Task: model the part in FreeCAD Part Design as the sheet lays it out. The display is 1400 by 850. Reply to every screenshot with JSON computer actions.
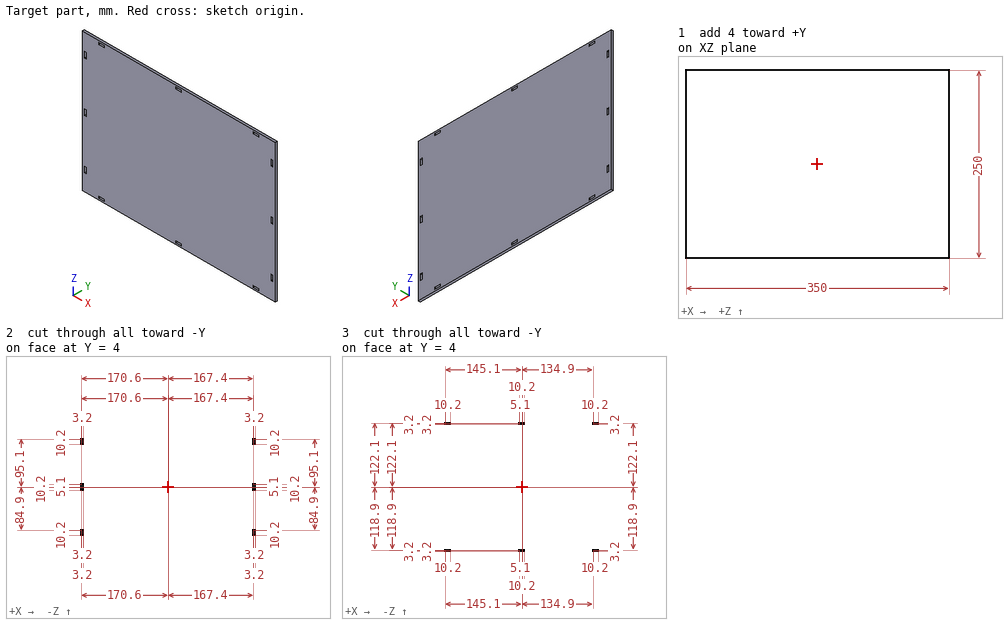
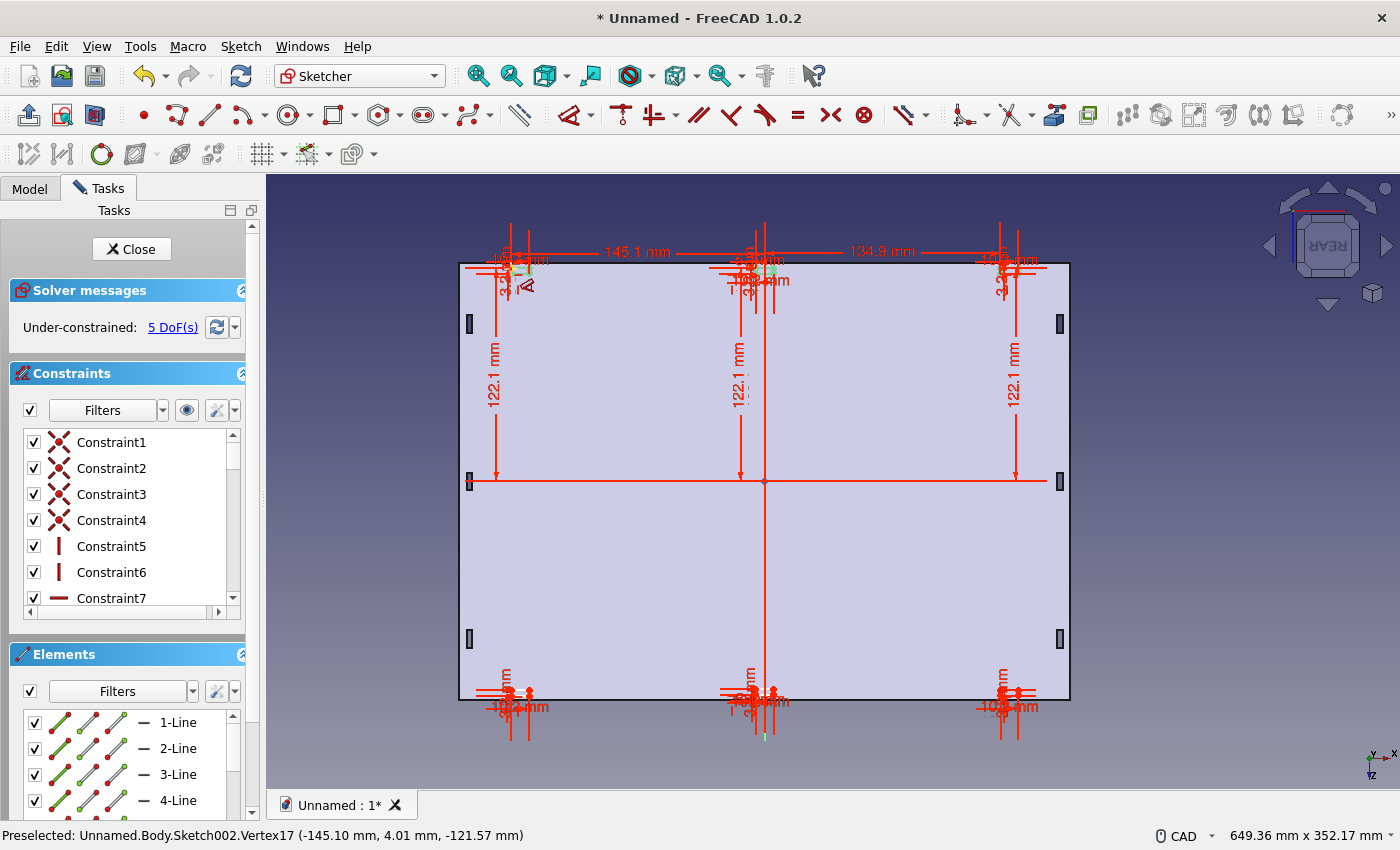
{"action": "scroll", "coordinate": [511, 690], "scroll_direction": "up", "scroll_amount": 4}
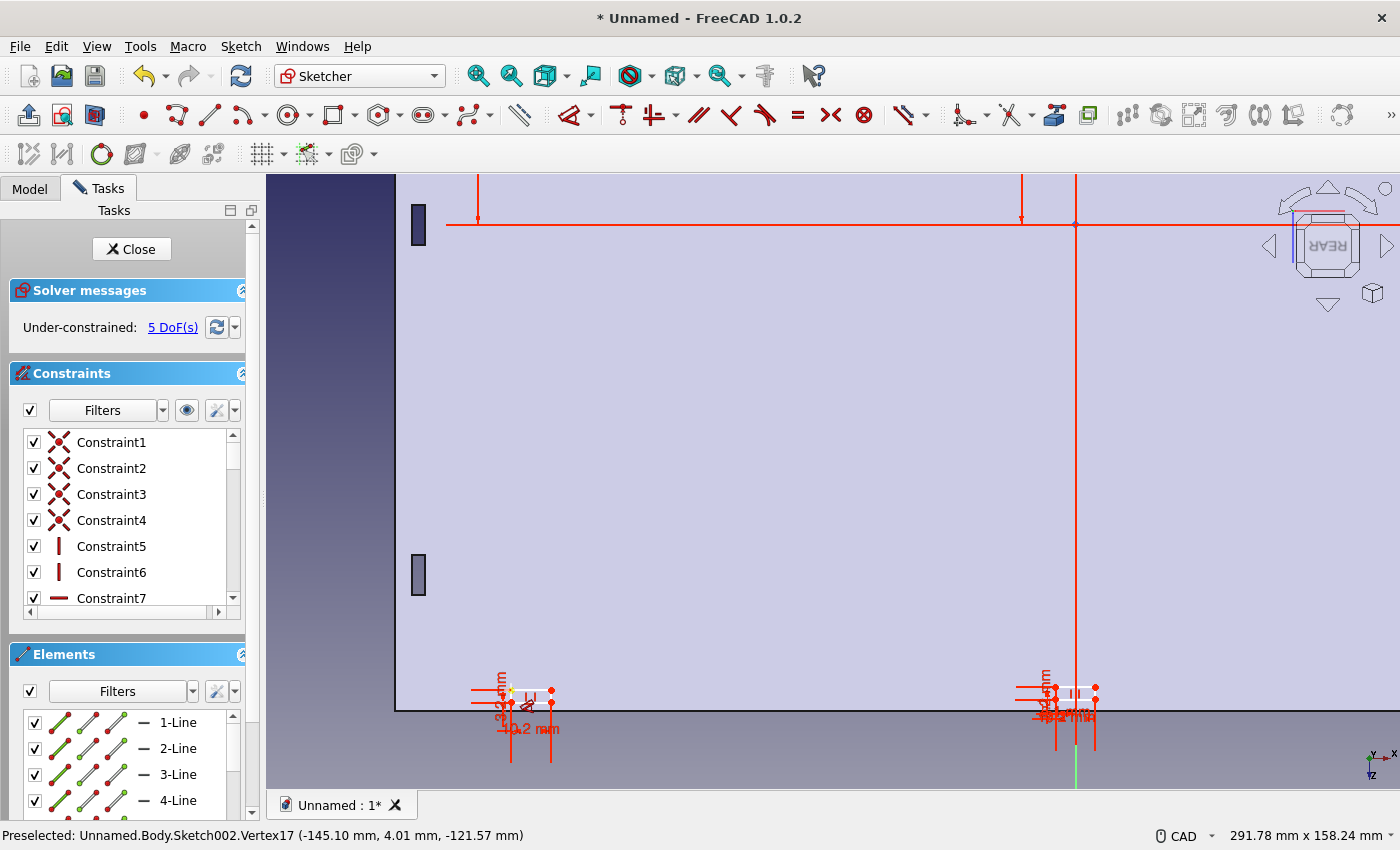
{"action": "left_click", "coordinate": [511, 690]}
{"action": "left_click", "coordinate": [793, 724]}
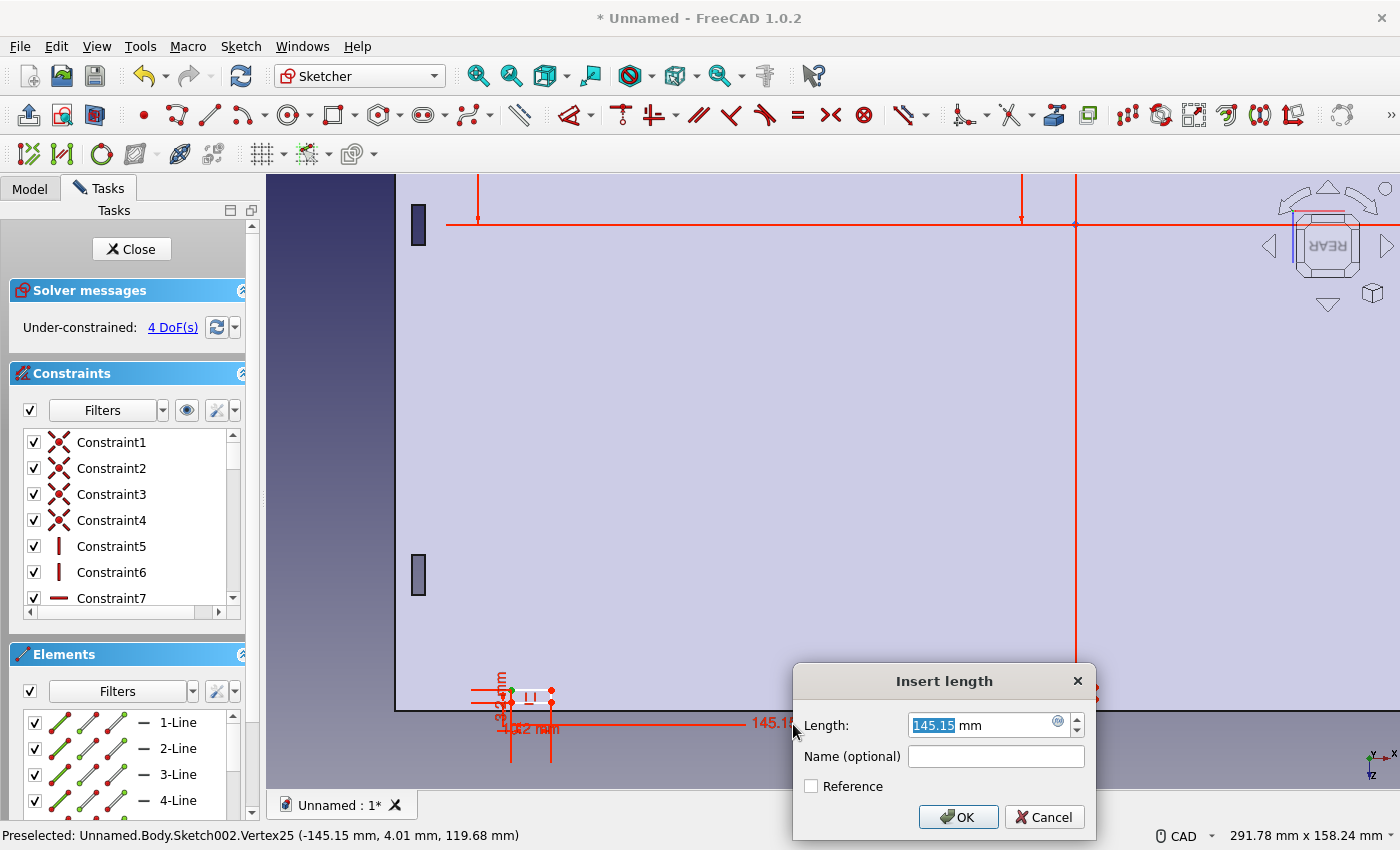
{"action": "type", "text": "145.1"}
{"action": "key", "text": "Return"}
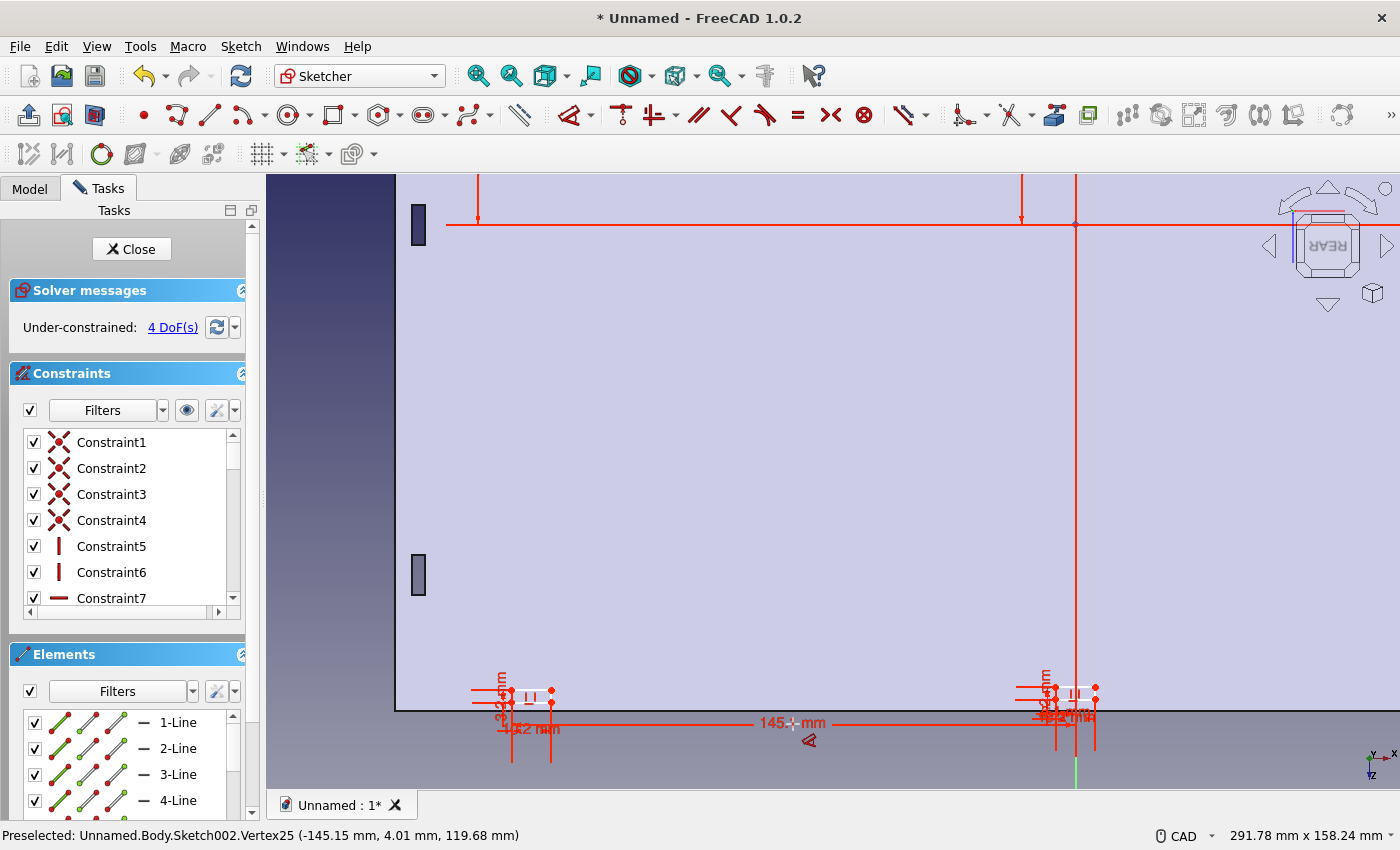
{"action": "left_click", "coordinate": [512, 690]}
{"action": "left_click", "coordinate": [478, 457]}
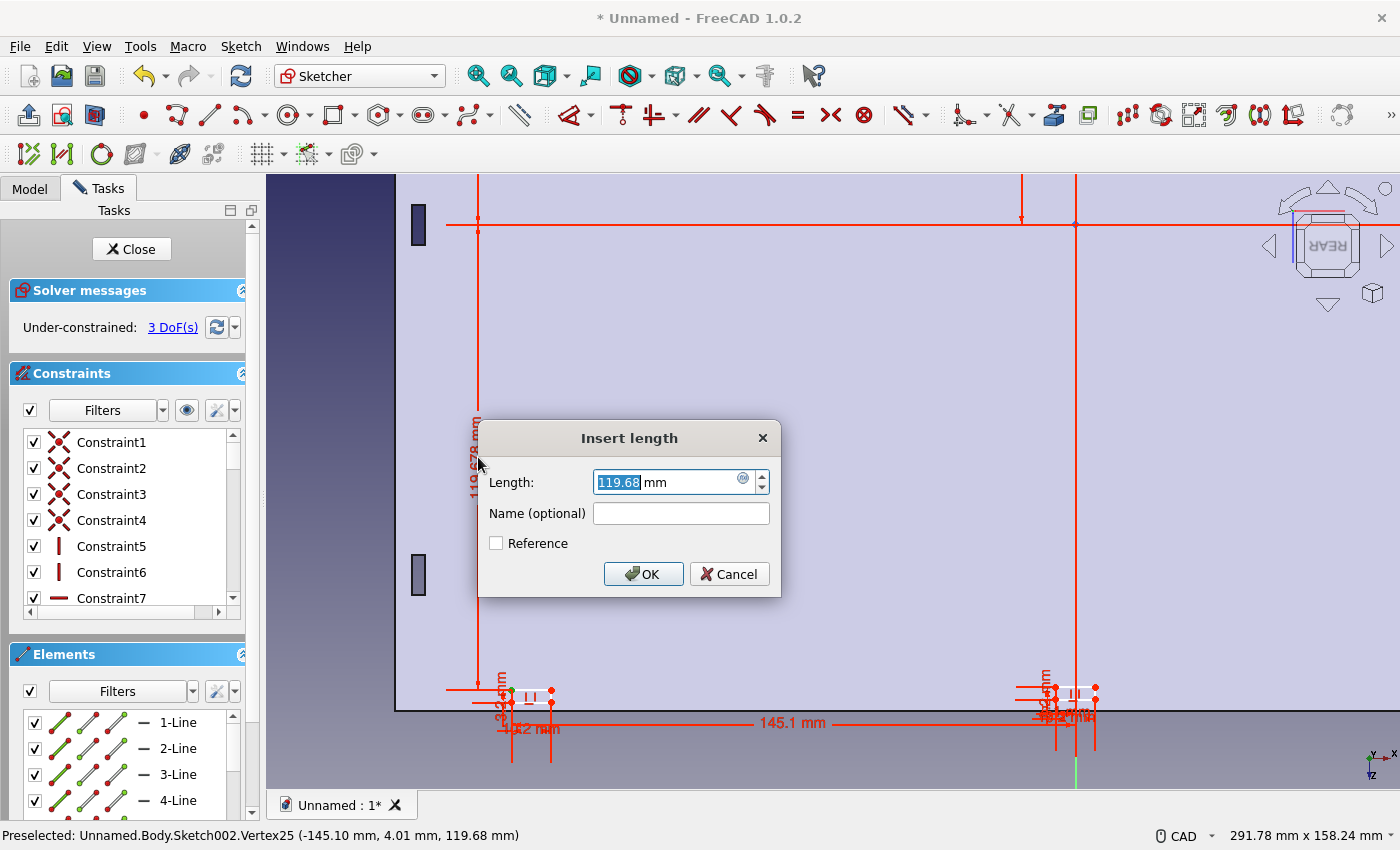
{"action": "type", "text": "118.9"}
{"action": "key", "text": "Return"}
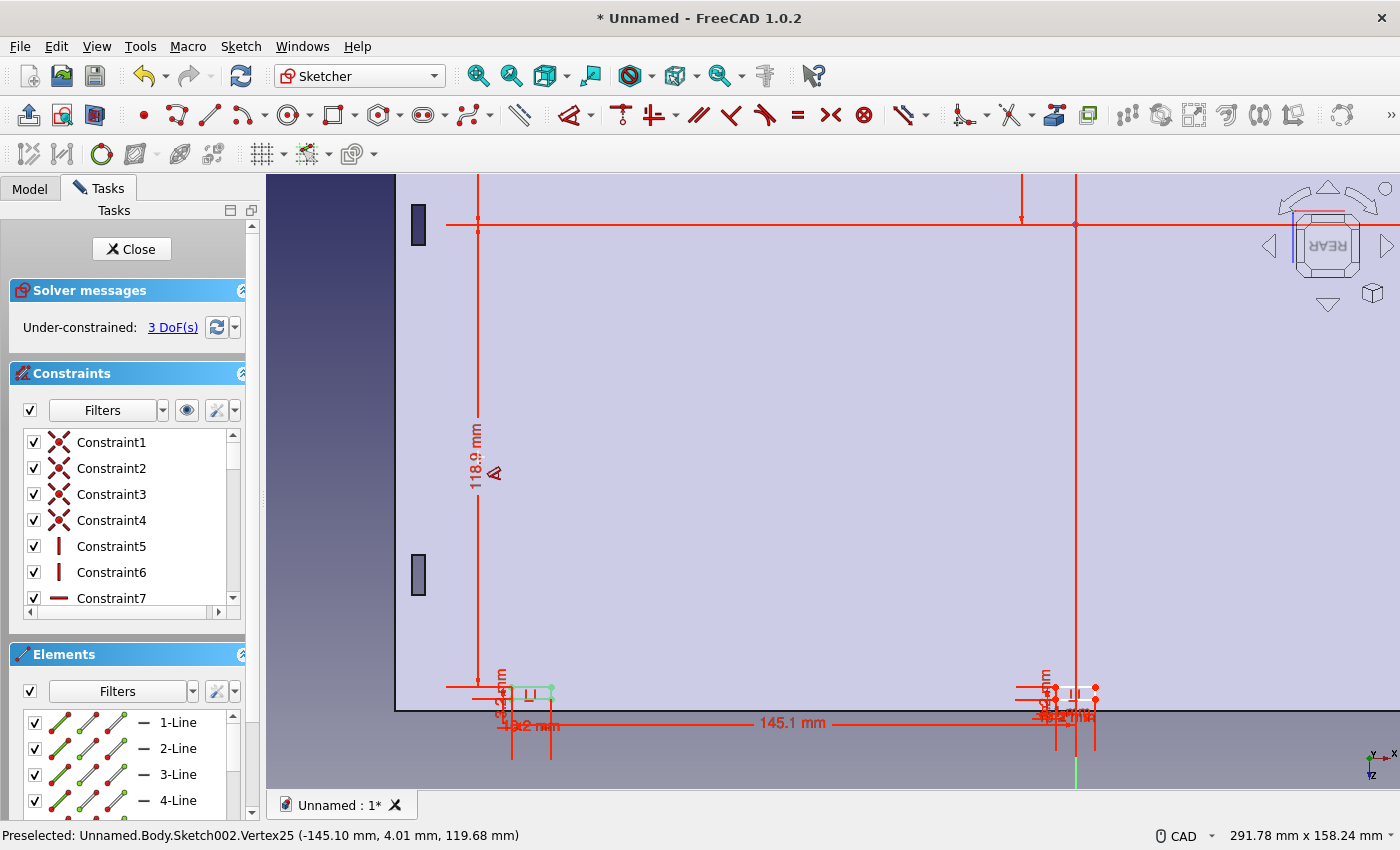
{"action": "scroll", "coordinate": [511, 691], "scroll_direction": "down", "scroll_amount": 4}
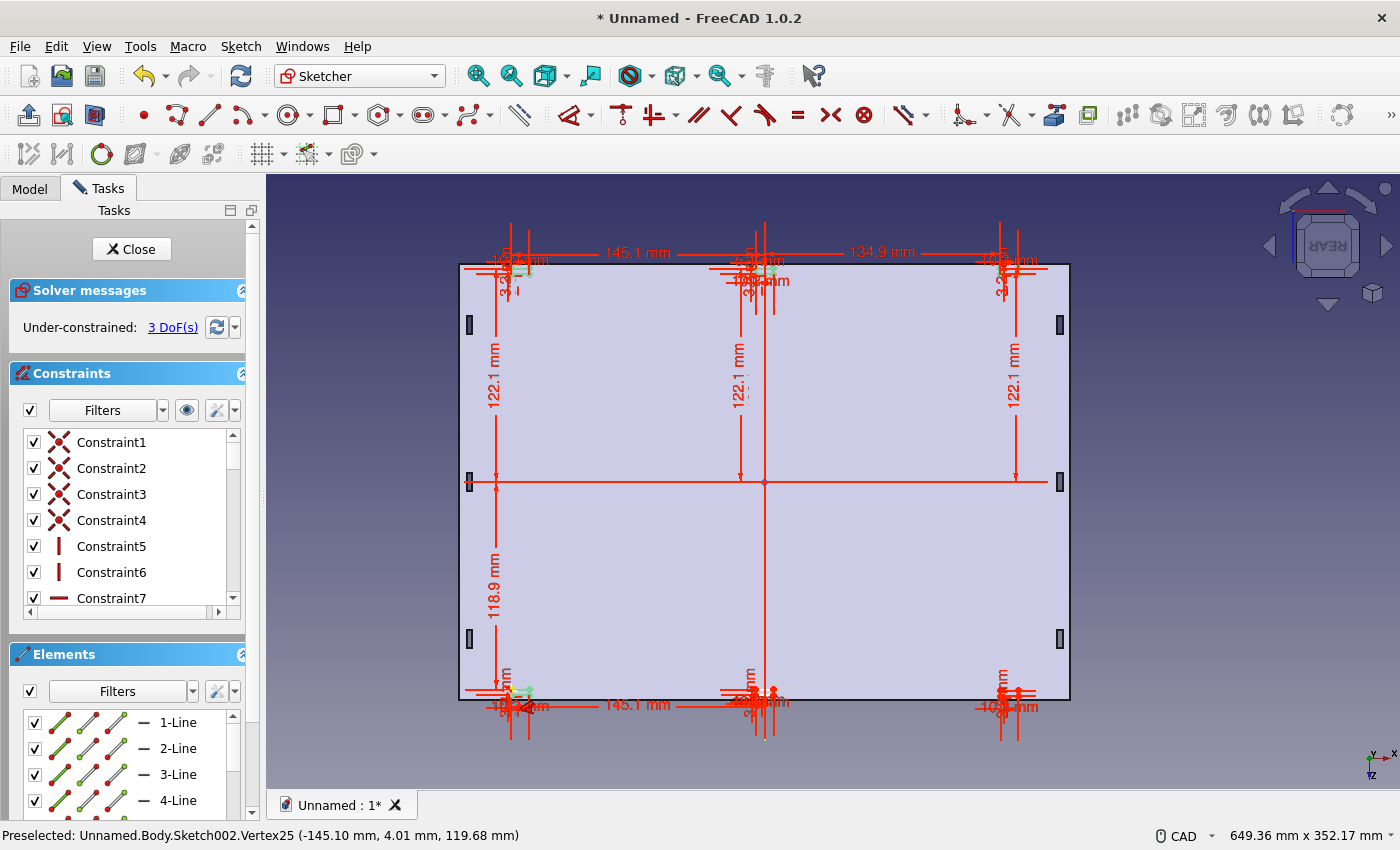
{"action": "scroll", "coordinate": [1001, 691], "scroll_direction": "up", "scroll_amount": 4}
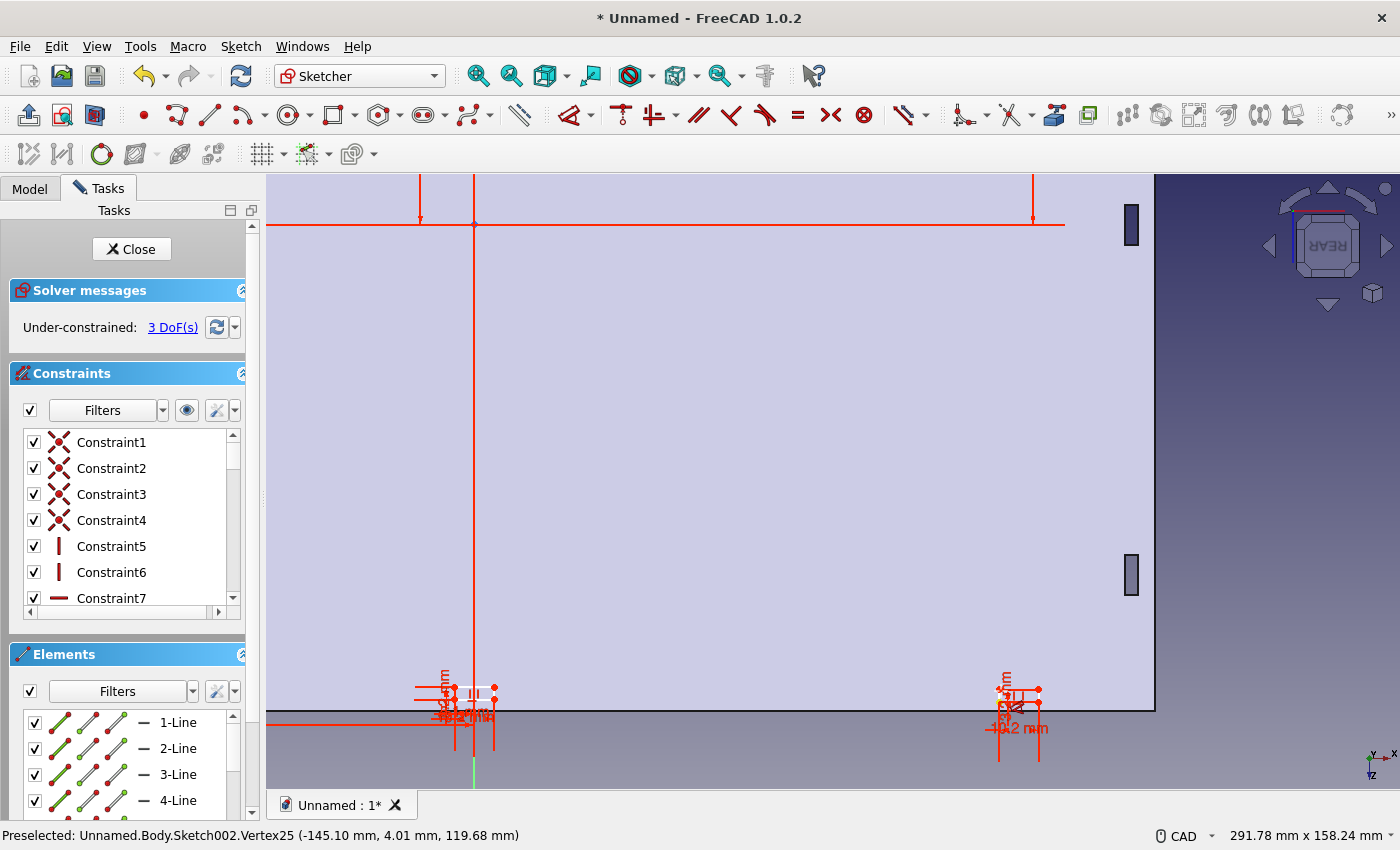
{"action": "left_click", "coordinate": [999, 690]}
{"action": "left_click", "coordinate": [737, 724]}